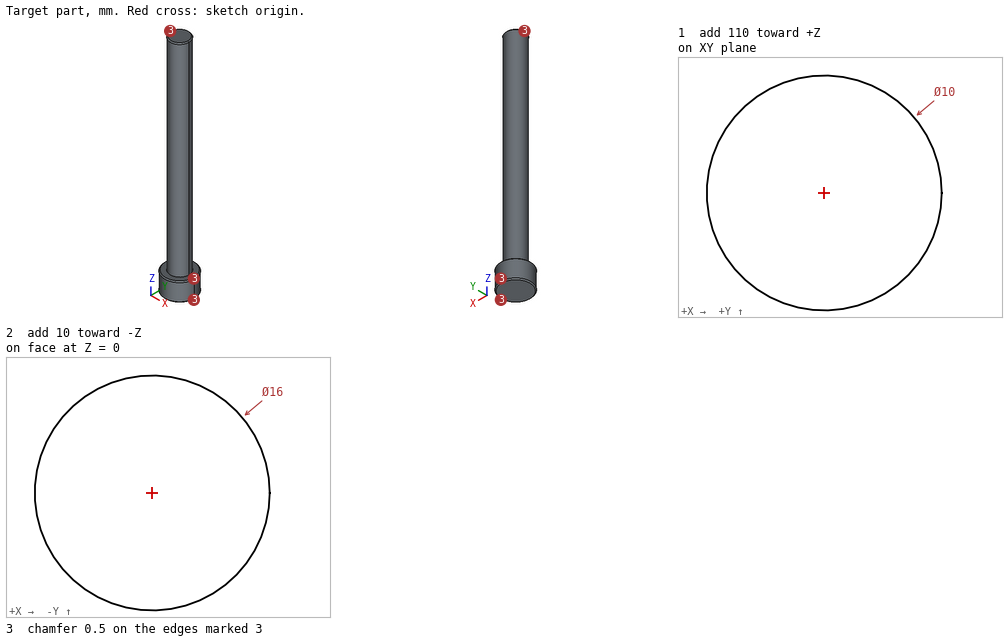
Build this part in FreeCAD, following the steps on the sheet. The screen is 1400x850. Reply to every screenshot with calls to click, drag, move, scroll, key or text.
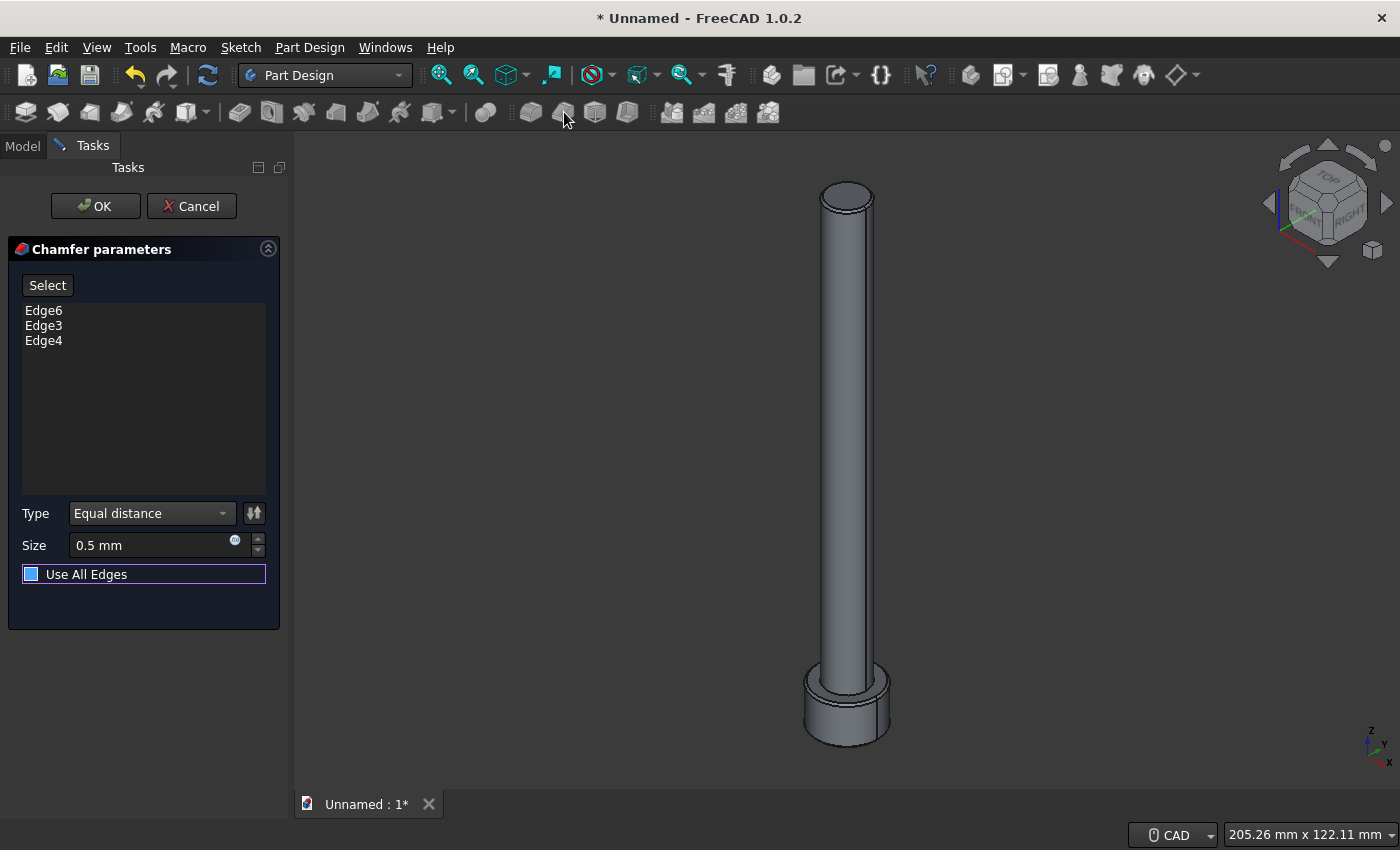
click(96, 206)